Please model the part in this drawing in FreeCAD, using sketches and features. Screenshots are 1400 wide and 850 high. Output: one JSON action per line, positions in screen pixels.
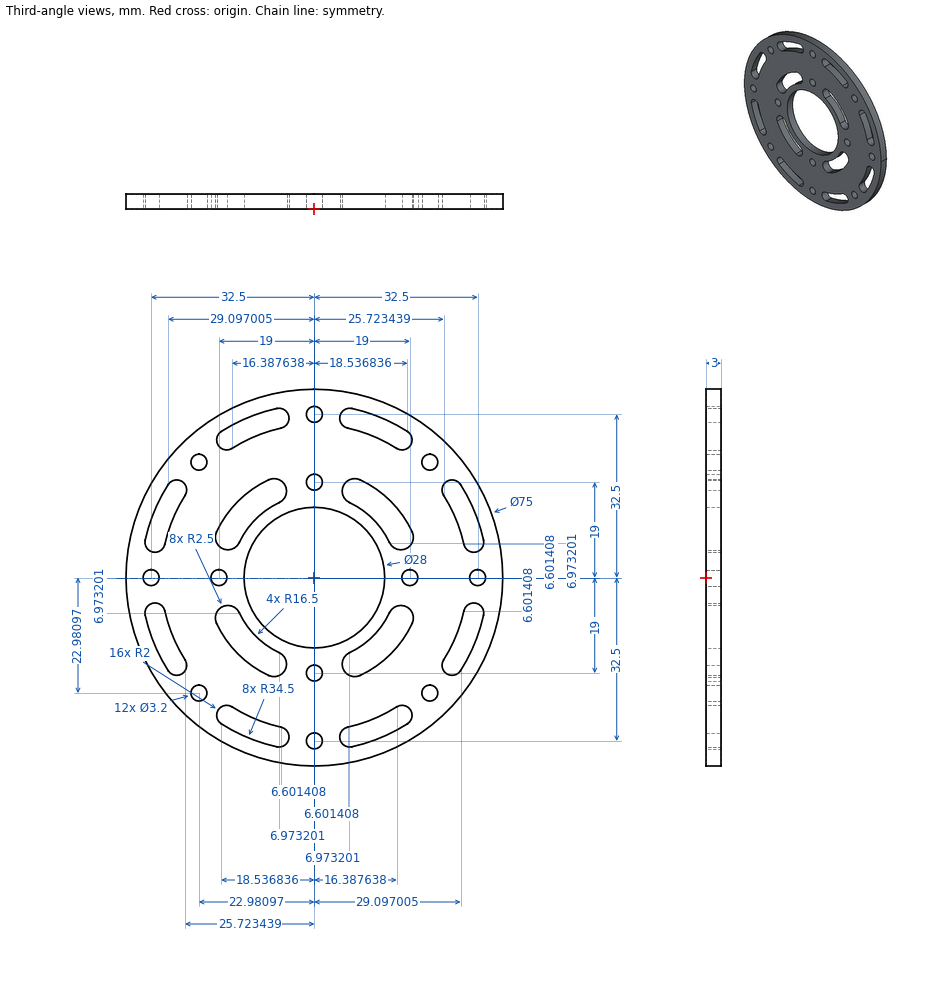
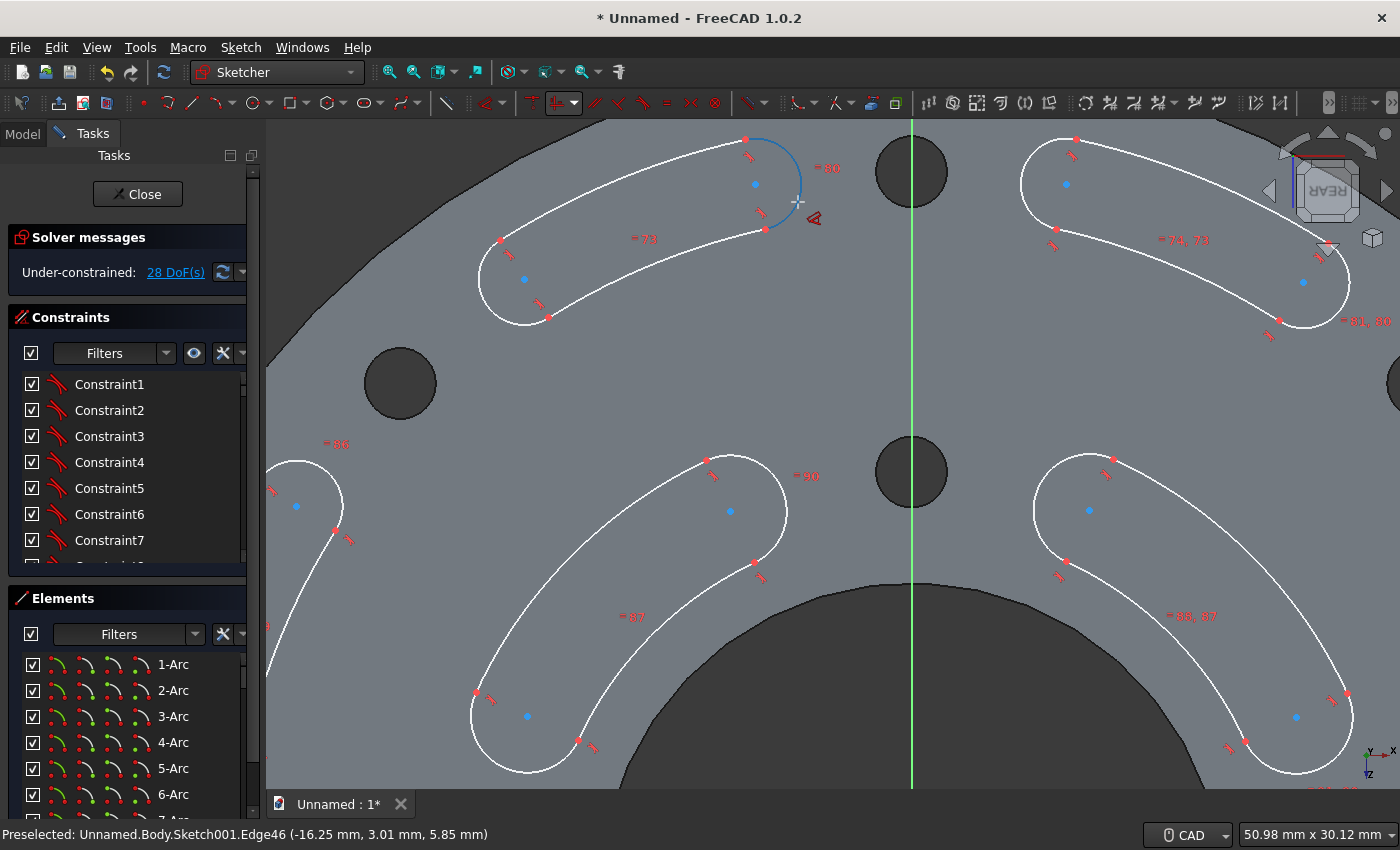
{"action": "left_click", "coordinate": [797, 203]}
{"action": "left_click", "coordinate": [826, 216]}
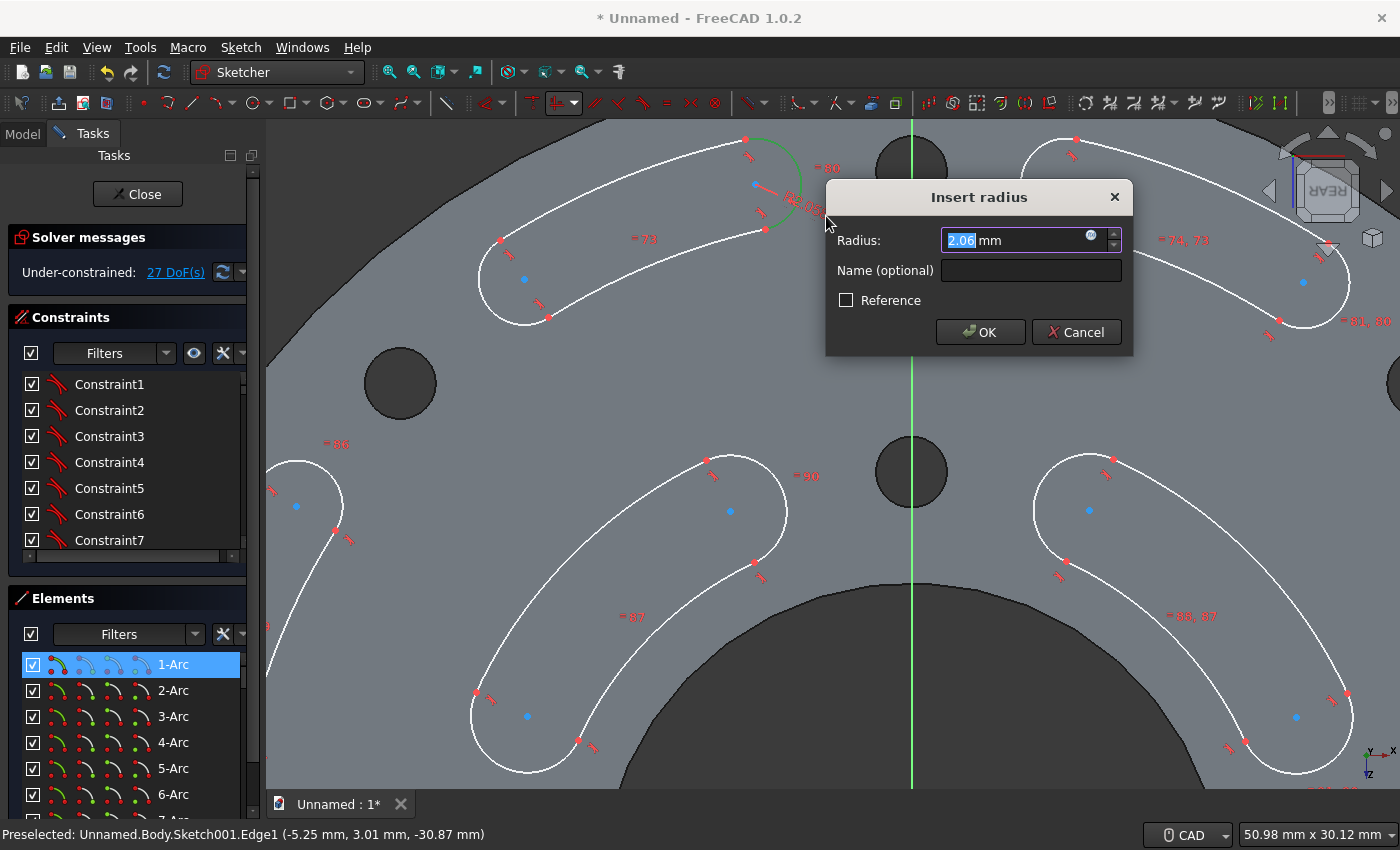
{"action": "type", "text": "2"}
{"action": "key", "text": "Return"}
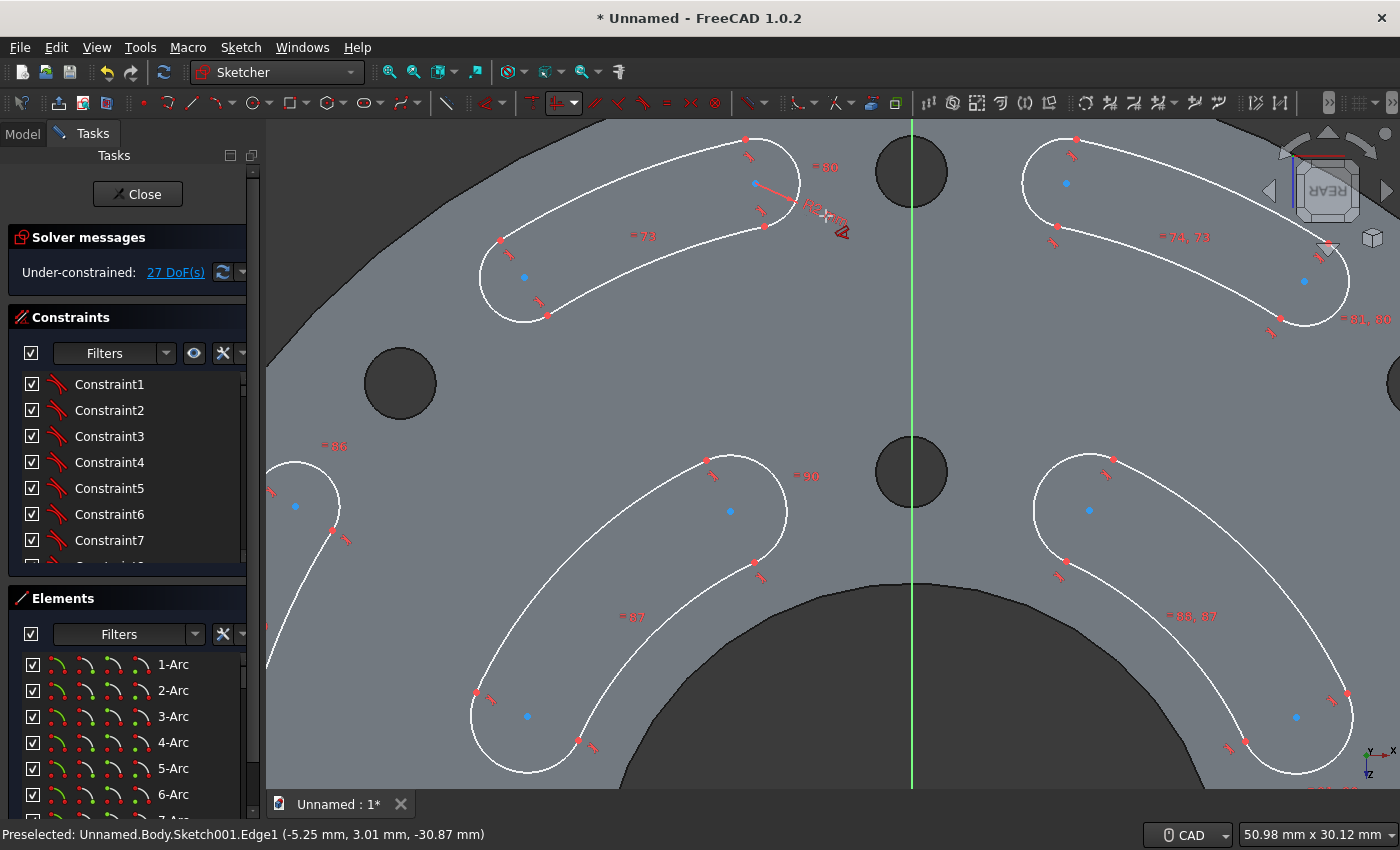
{"action": "left_click", "coordinate": [669, 161]}
{"action": "left_click", "coordinate": [324, 345]}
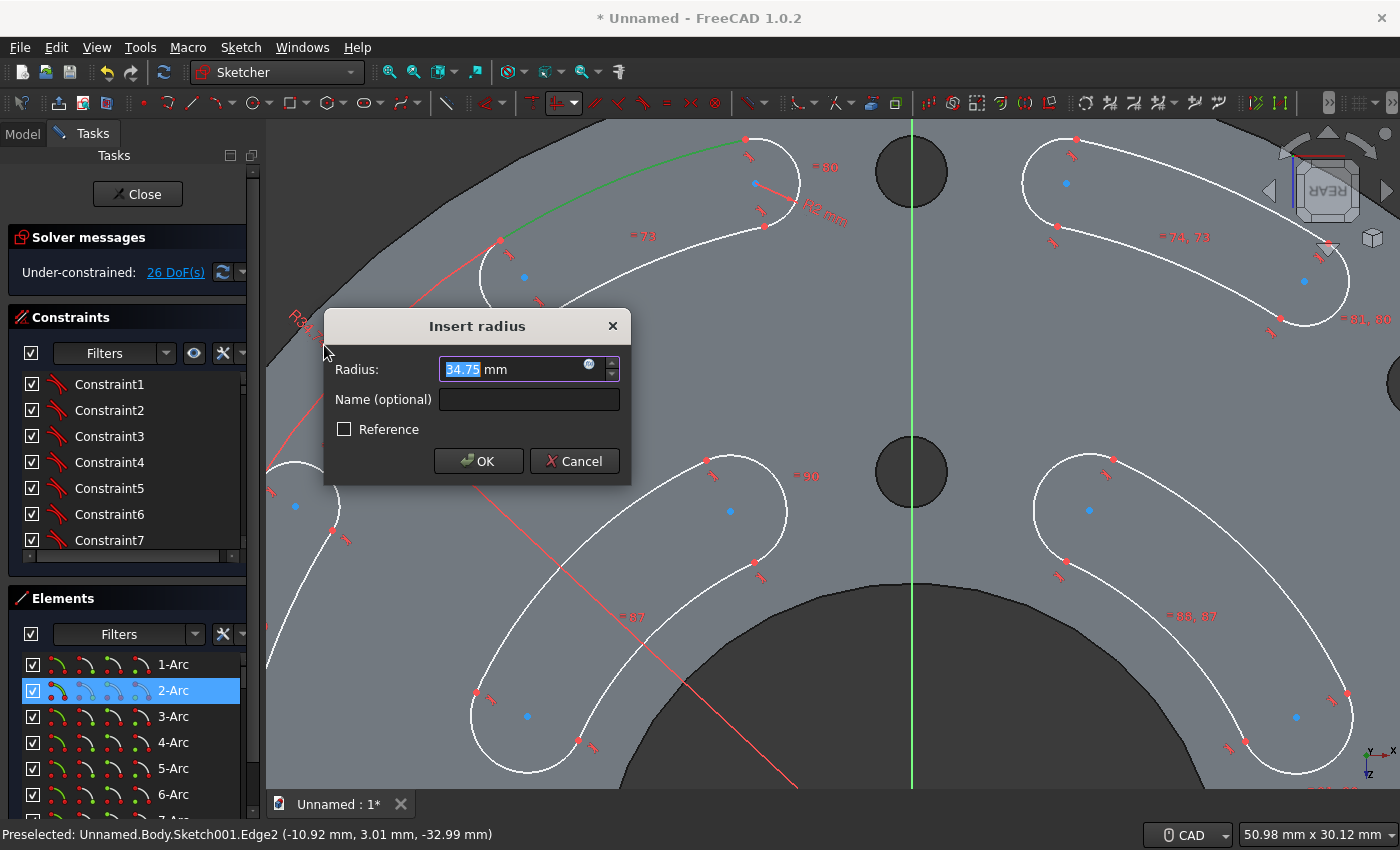
{"action": "type", "text": "34.5"}
{"action": "key", "text": "Return"}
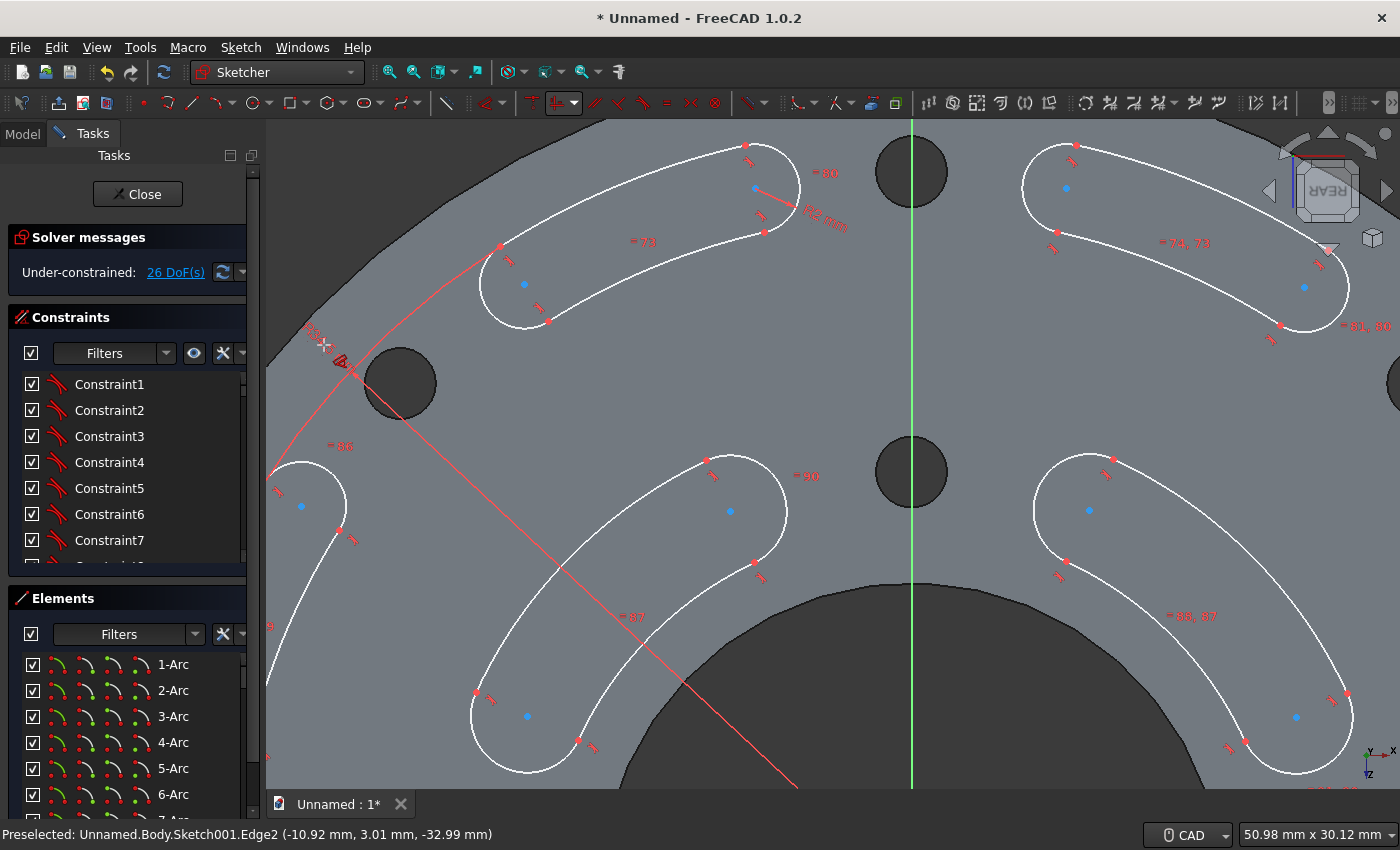
{"action": "left_click", "coordinate": [689, 602]}
{"action": "left_click", "coordinate": [670, 577]}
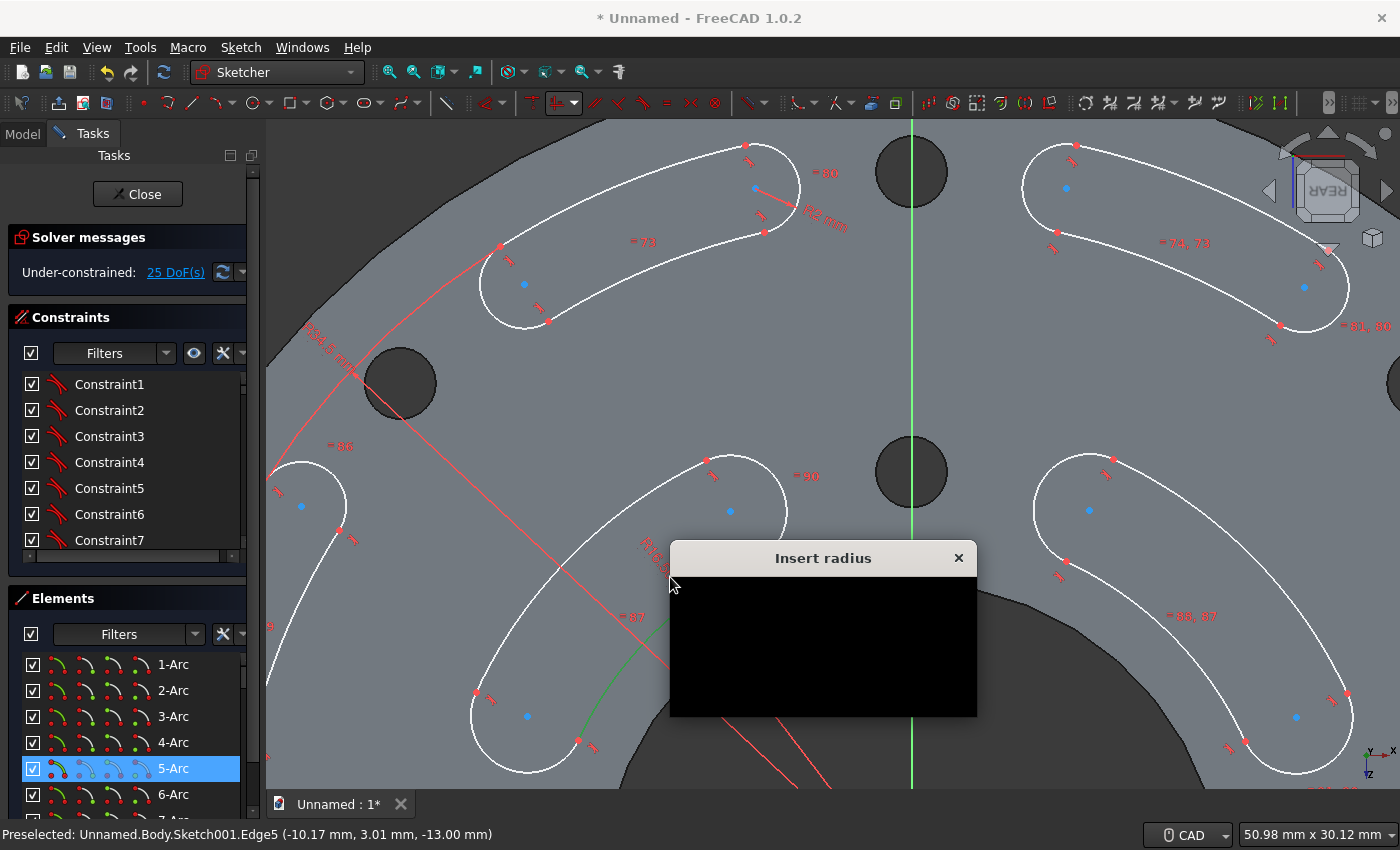
{"action": "type", "text": "16.5"}
{"action": "key", "text": "Return"}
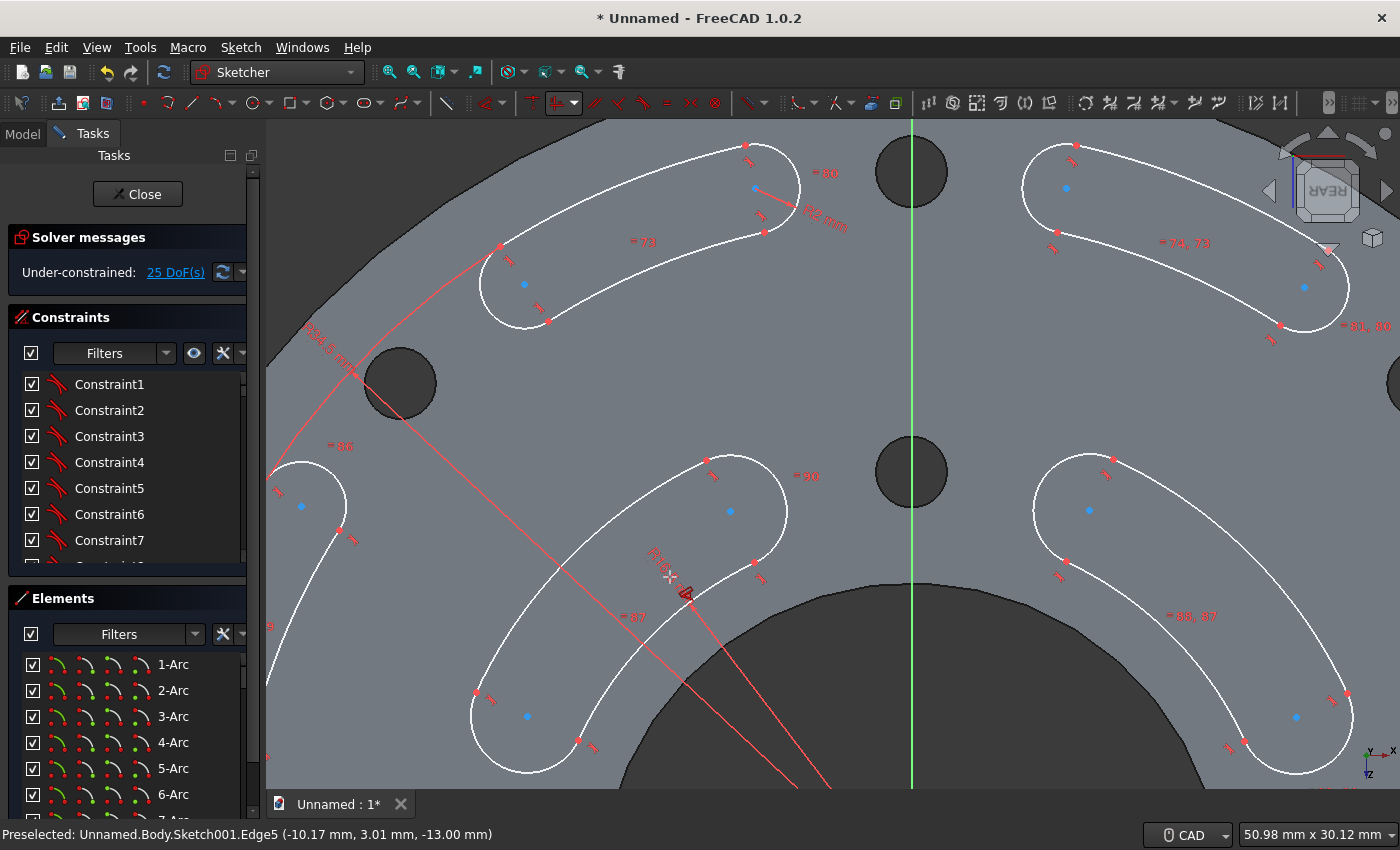
{"action": "left_click", "coordinate": [786, 522]}
{"action": "left_click", "coordinate": [817, 528]}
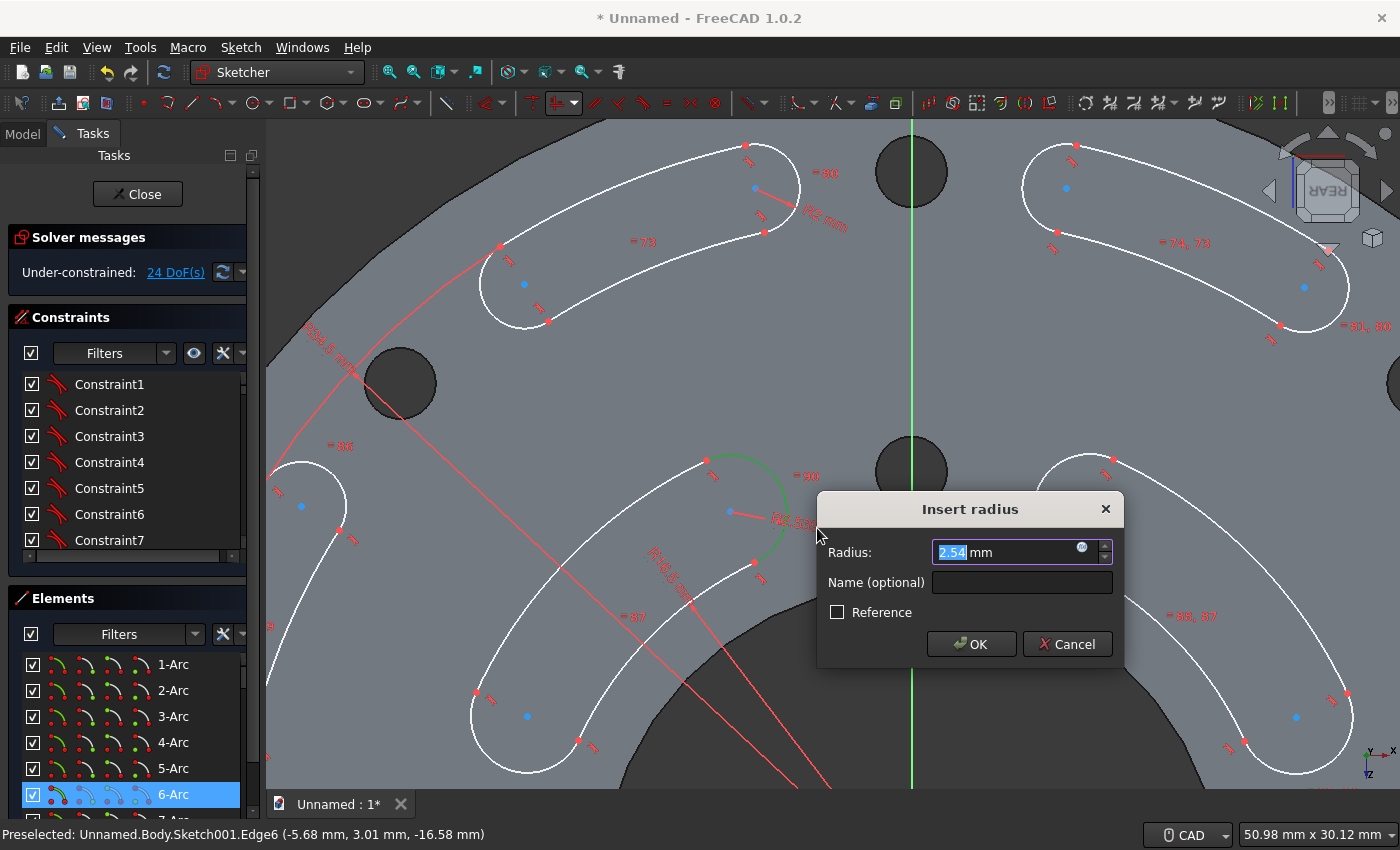
{"action": "type", "text": "2.5"}
{"action": "key", "text": "Return"}